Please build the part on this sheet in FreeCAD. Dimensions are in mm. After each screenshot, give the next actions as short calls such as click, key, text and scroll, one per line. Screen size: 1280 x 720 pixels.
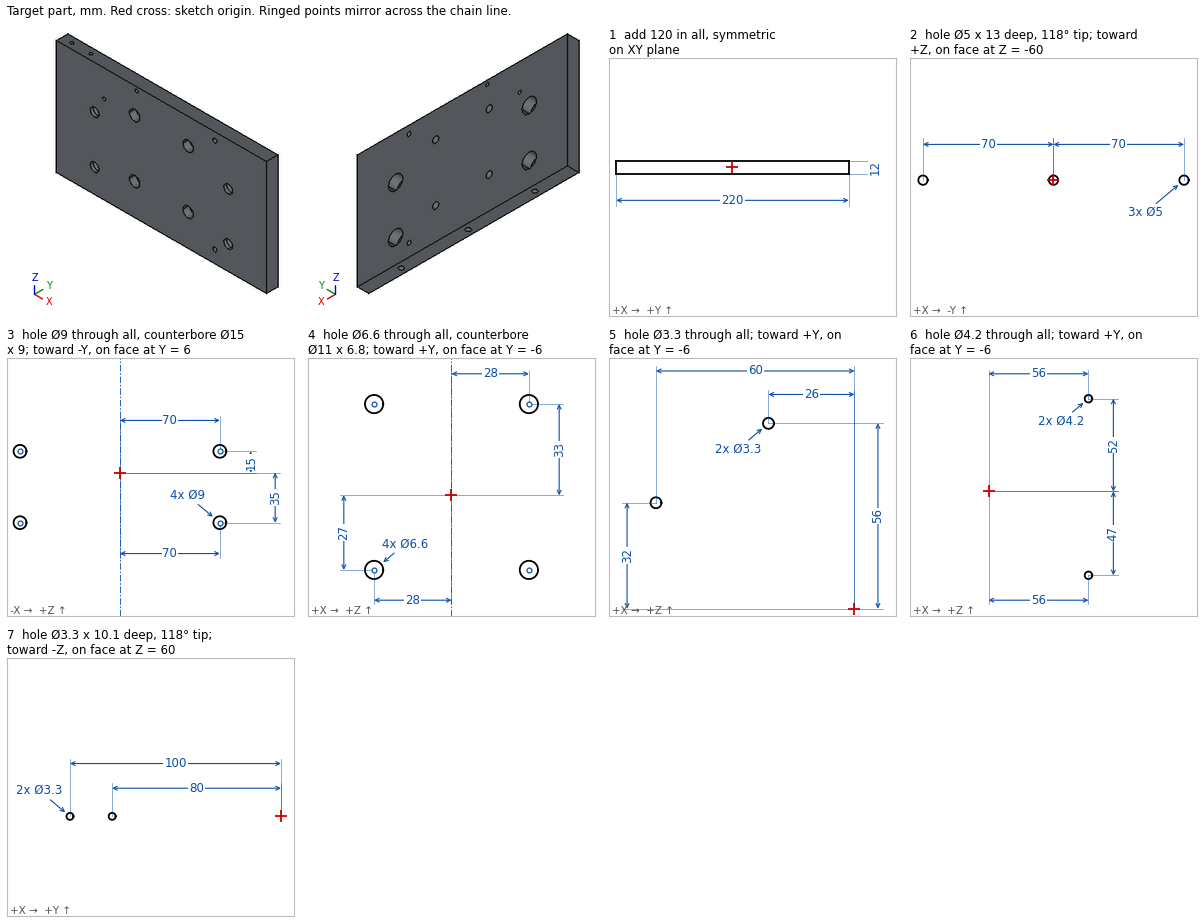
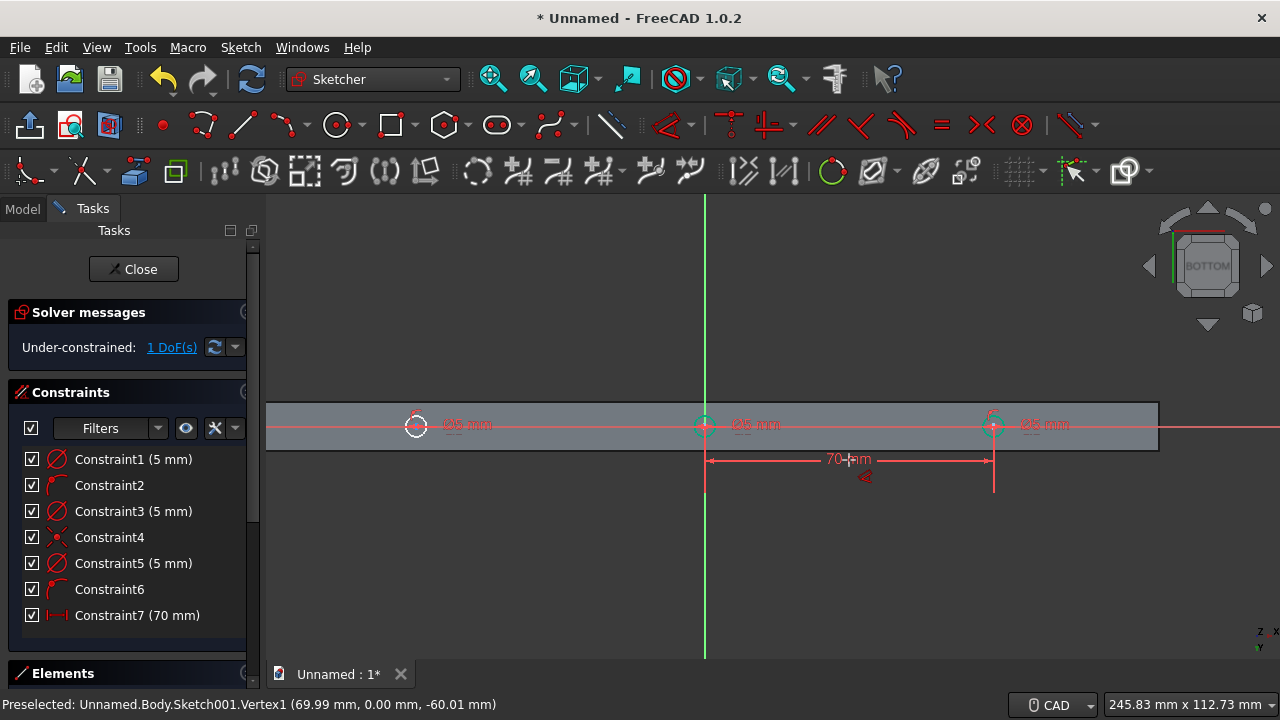
click(416, 426)
click(560, 460)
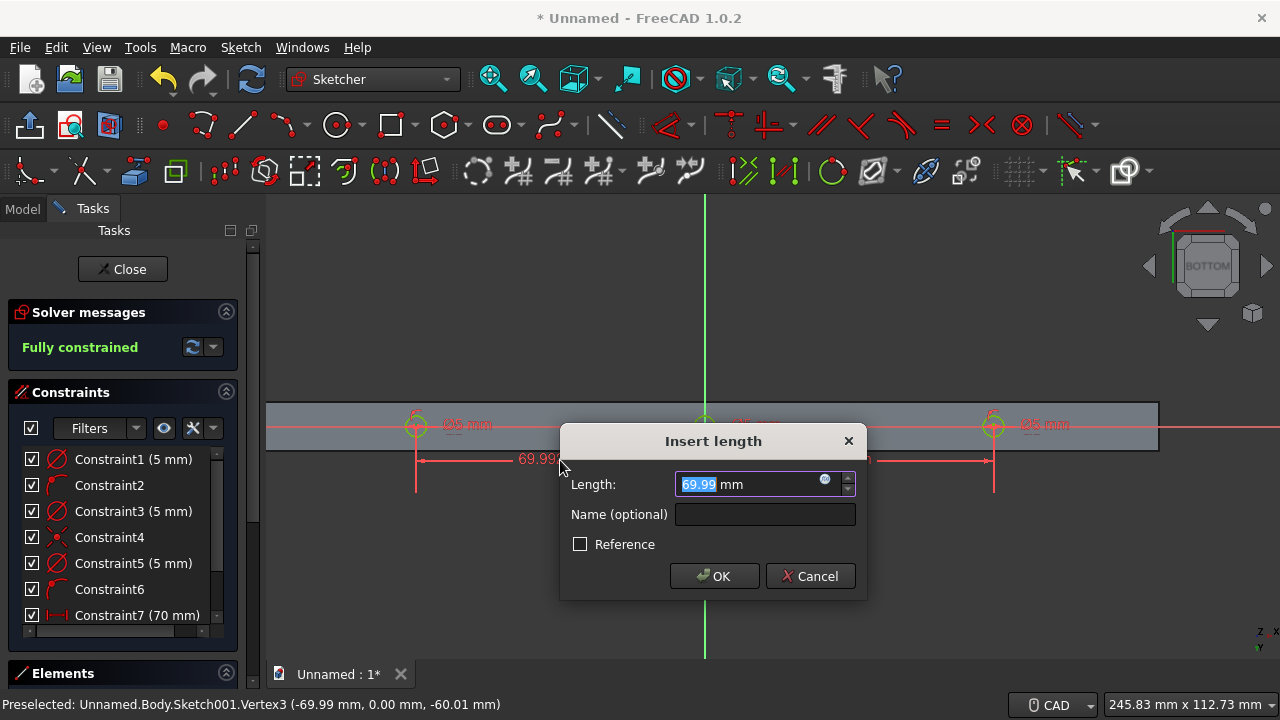
text(70)
key(Return)
key(Escape)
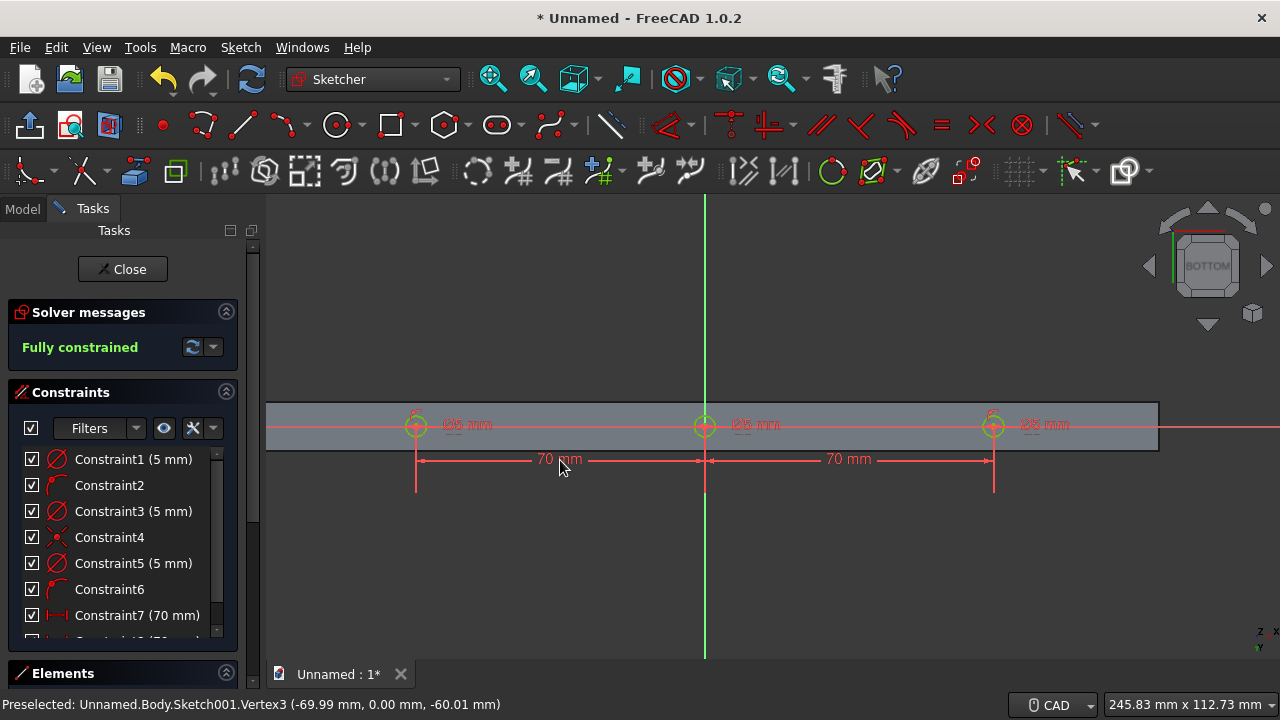
click(123, 269)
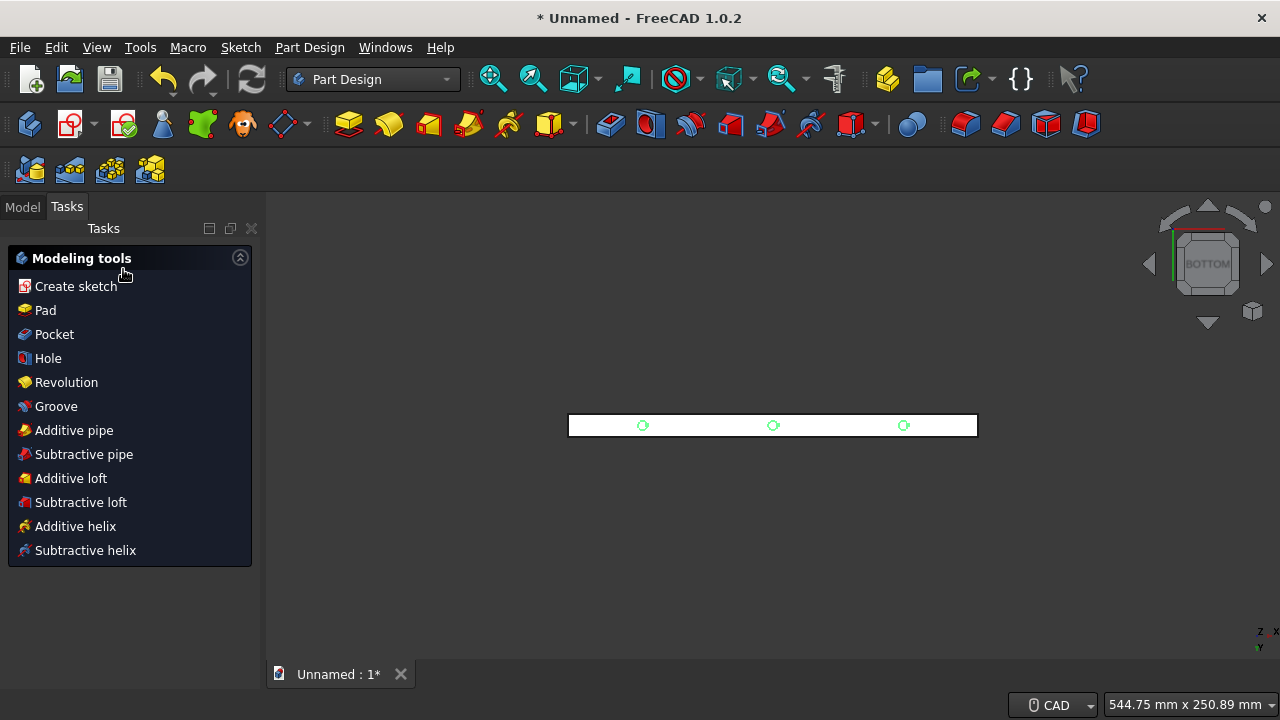
click(652, 124)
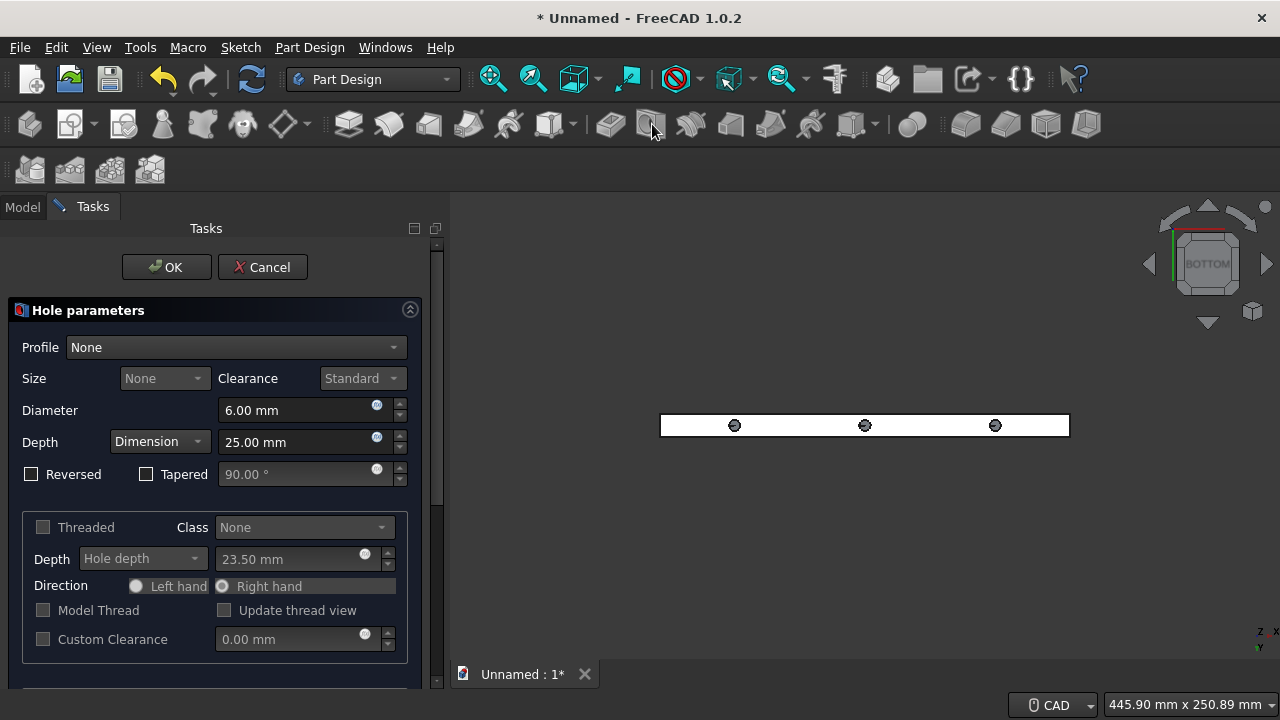
triple_click(305, 410)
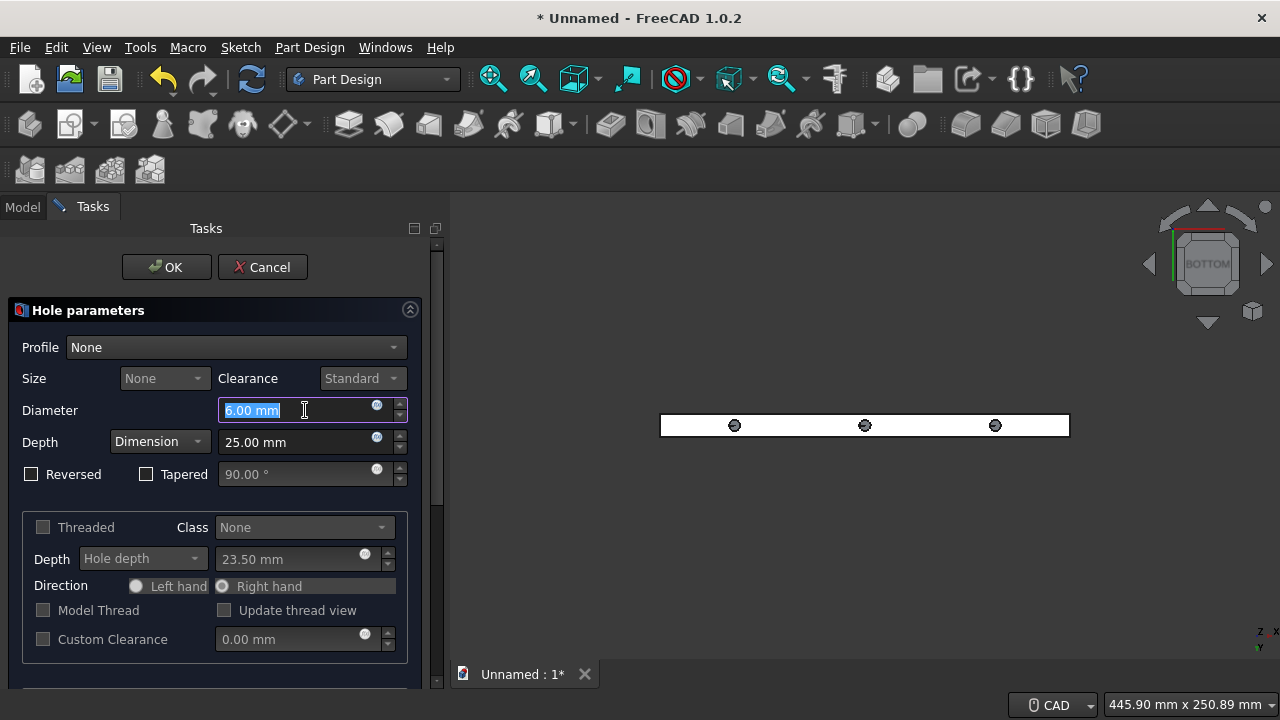
text(5)
key(Tab)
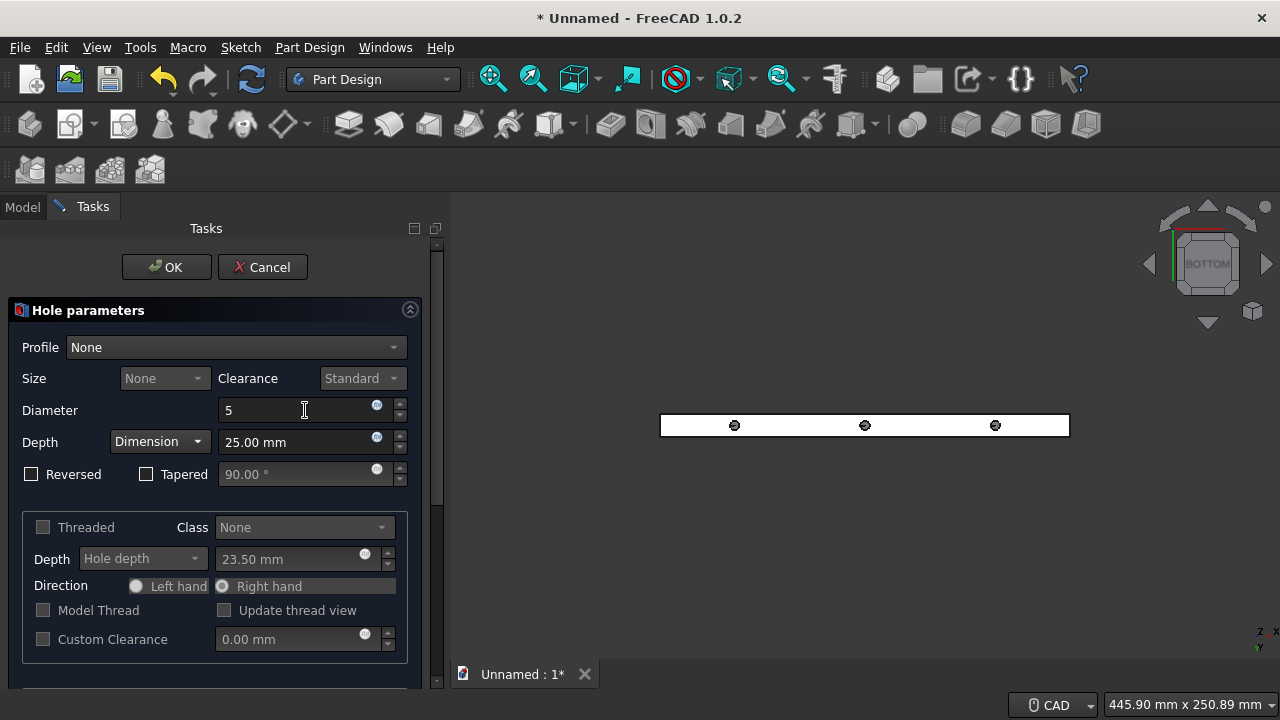
triple_click(305, 442)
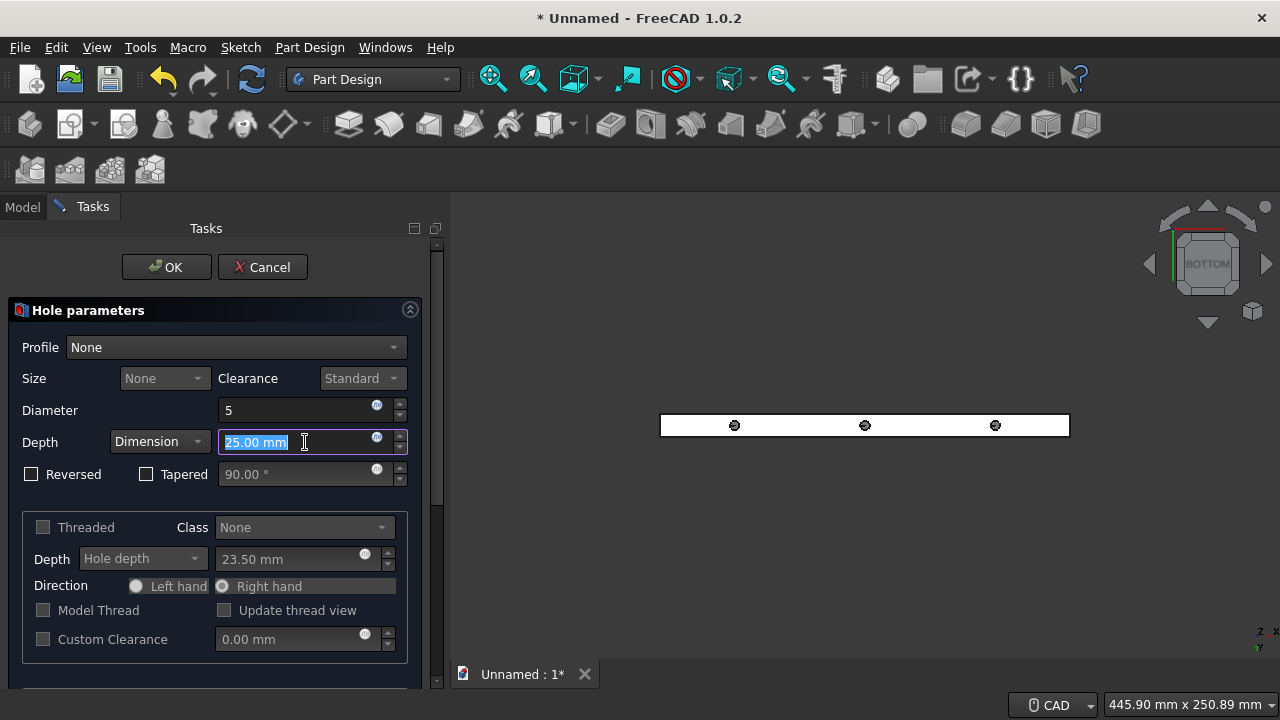
text(13)
key(Tab)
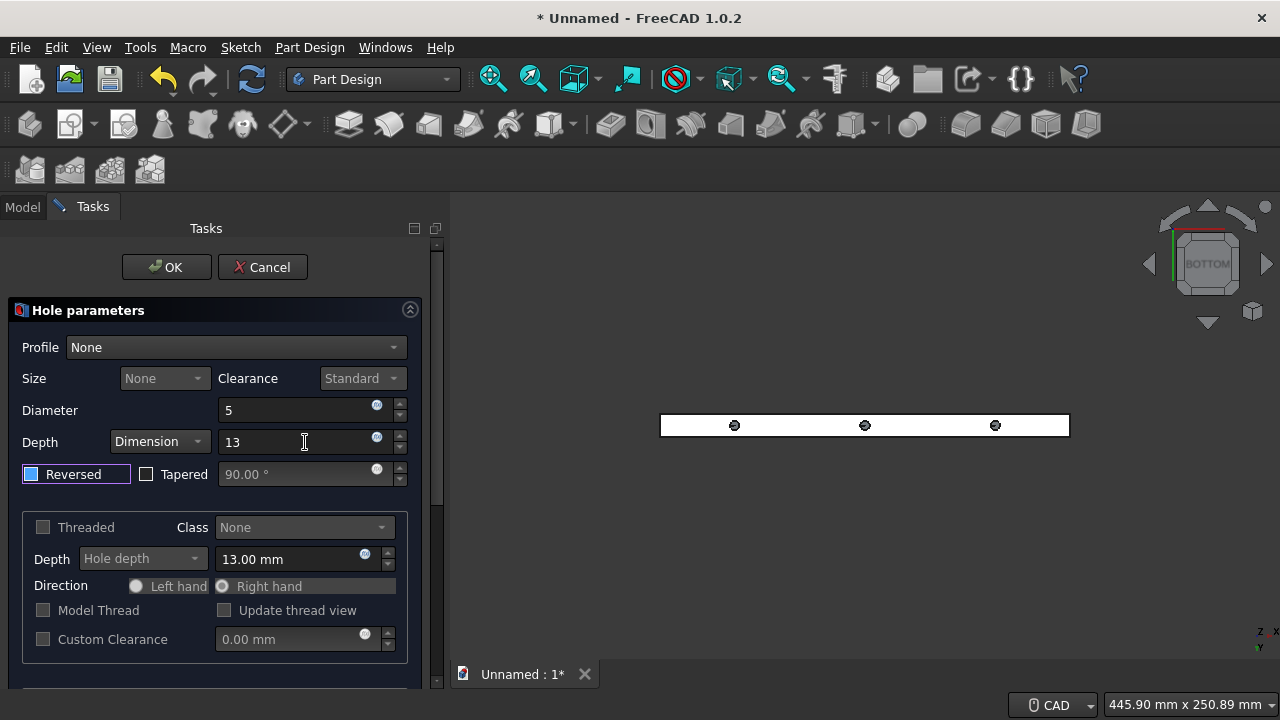
click(167, 267)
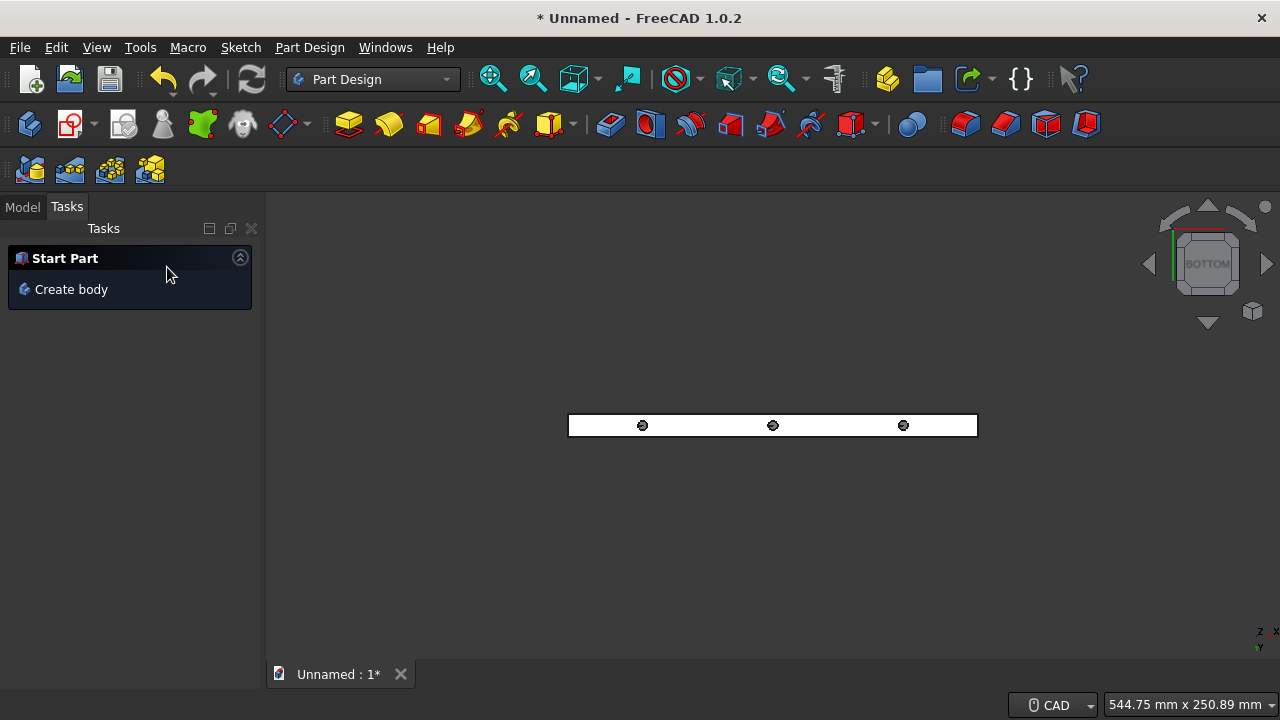
click(494, 80)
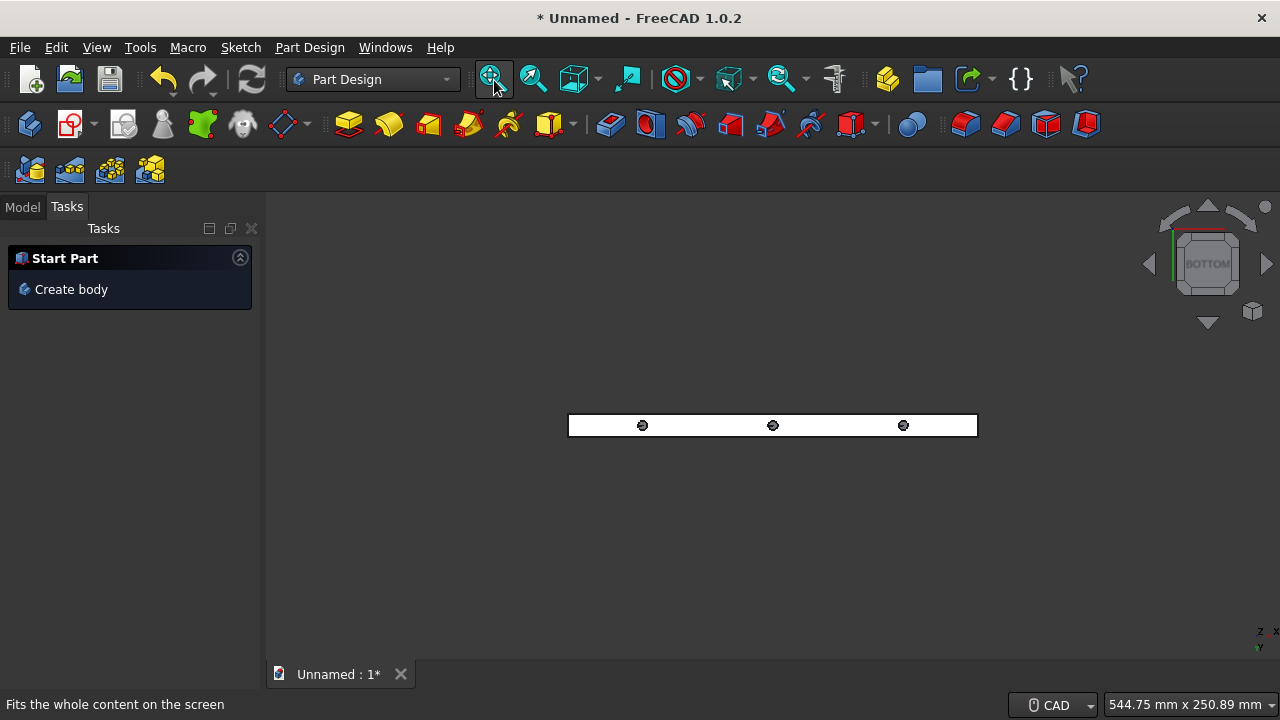
key(4)